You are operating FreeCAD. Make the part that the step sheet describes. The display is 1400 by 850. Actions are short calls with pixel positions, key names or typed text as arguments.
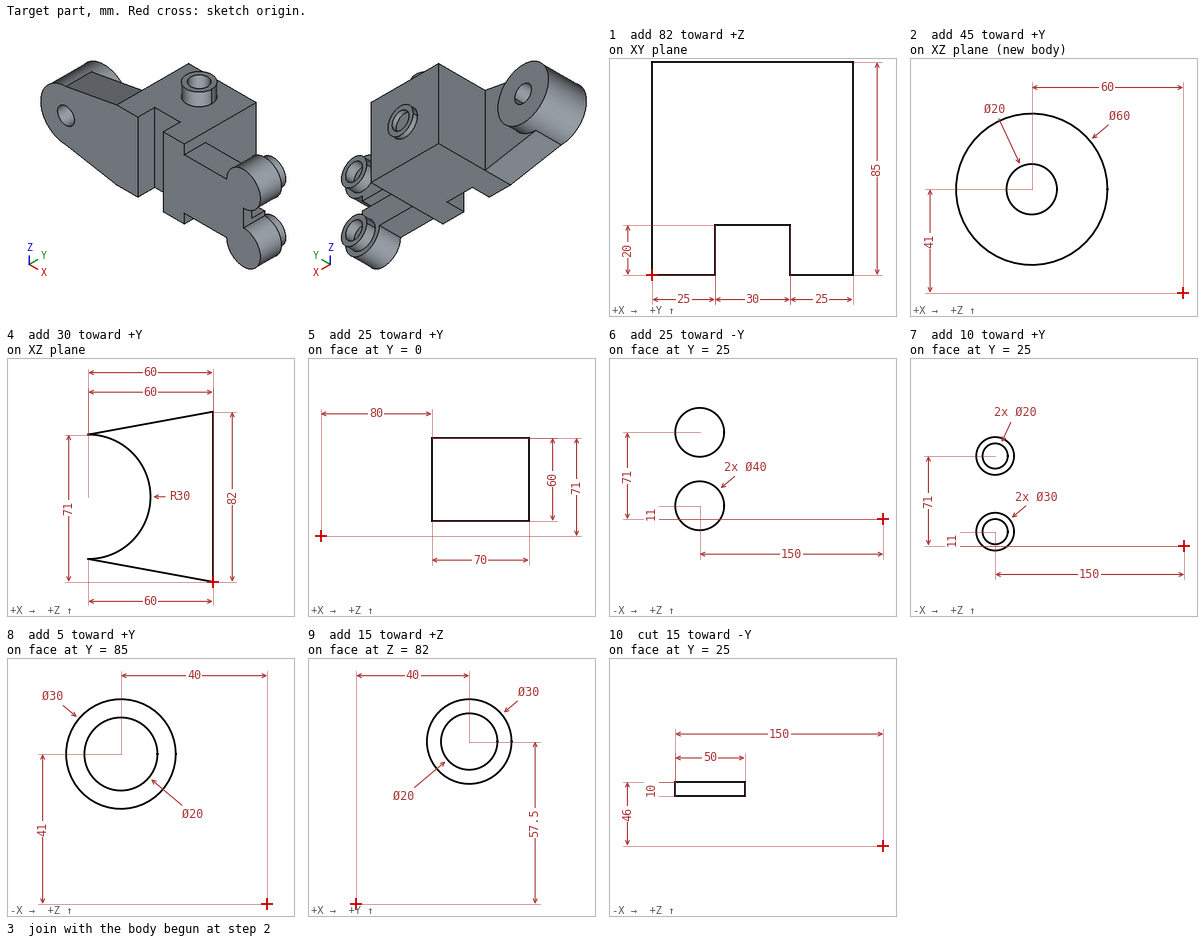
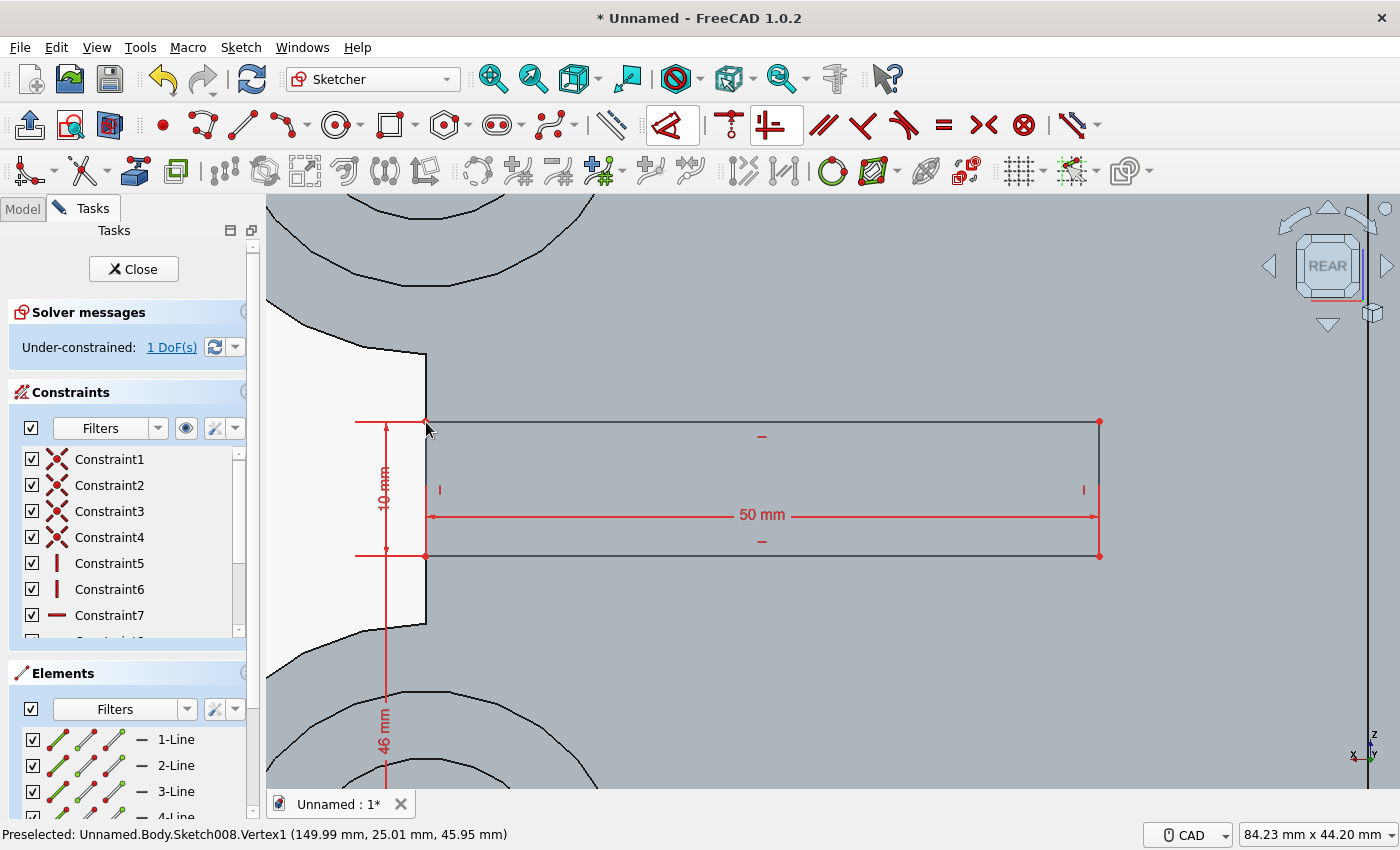
click(426, 422)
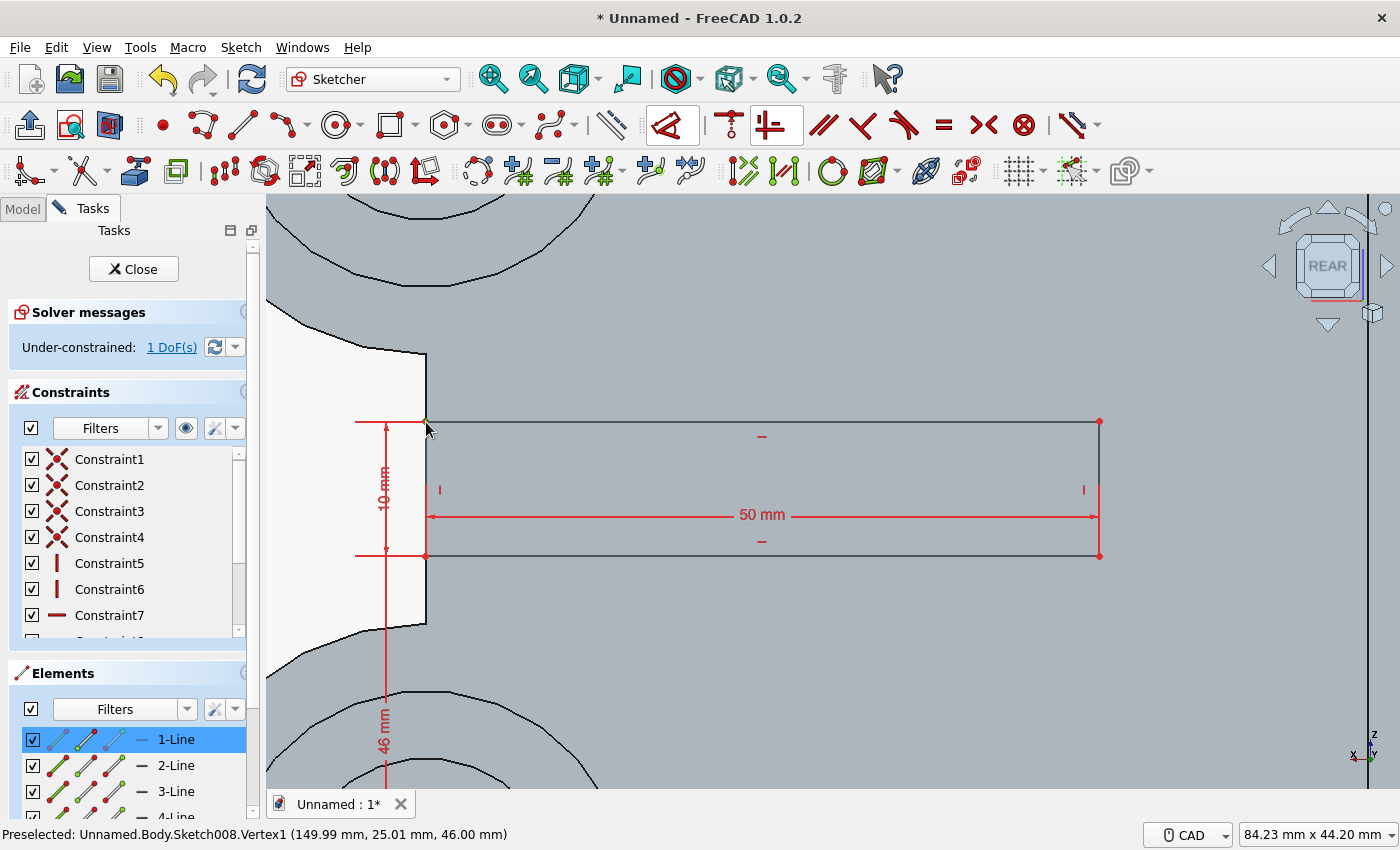
key(l)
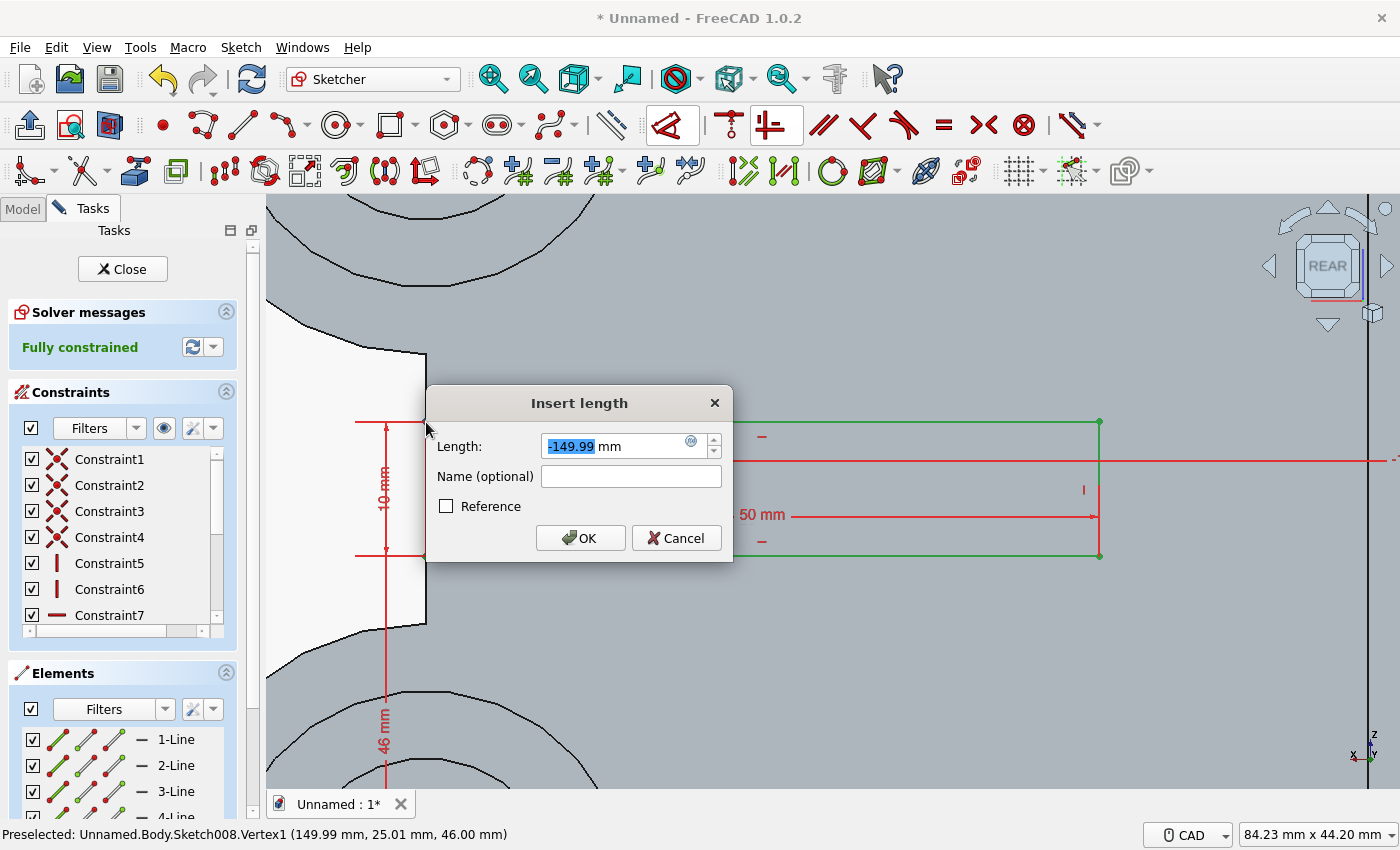
text(-150)
key(Return)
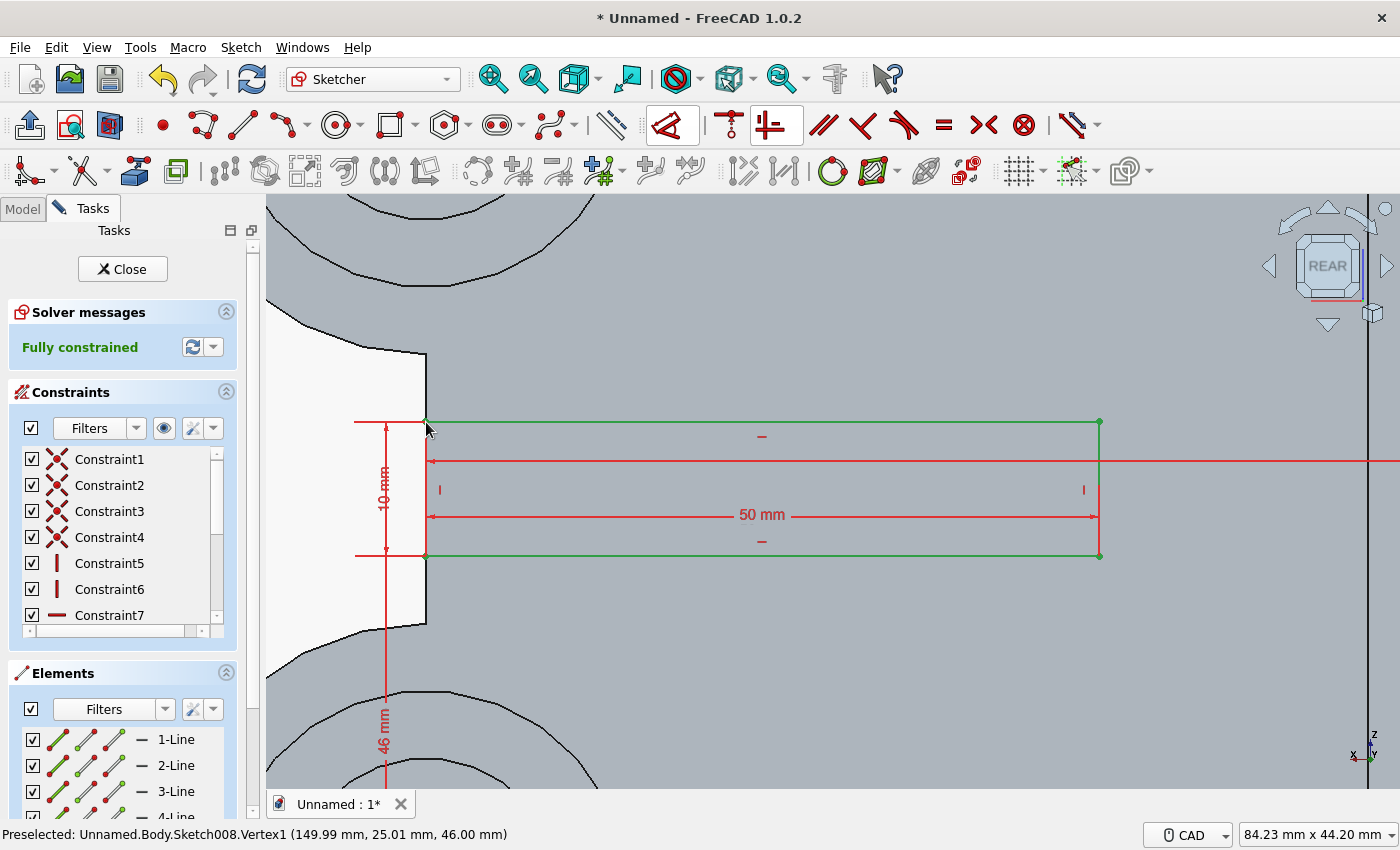
click(123, 269)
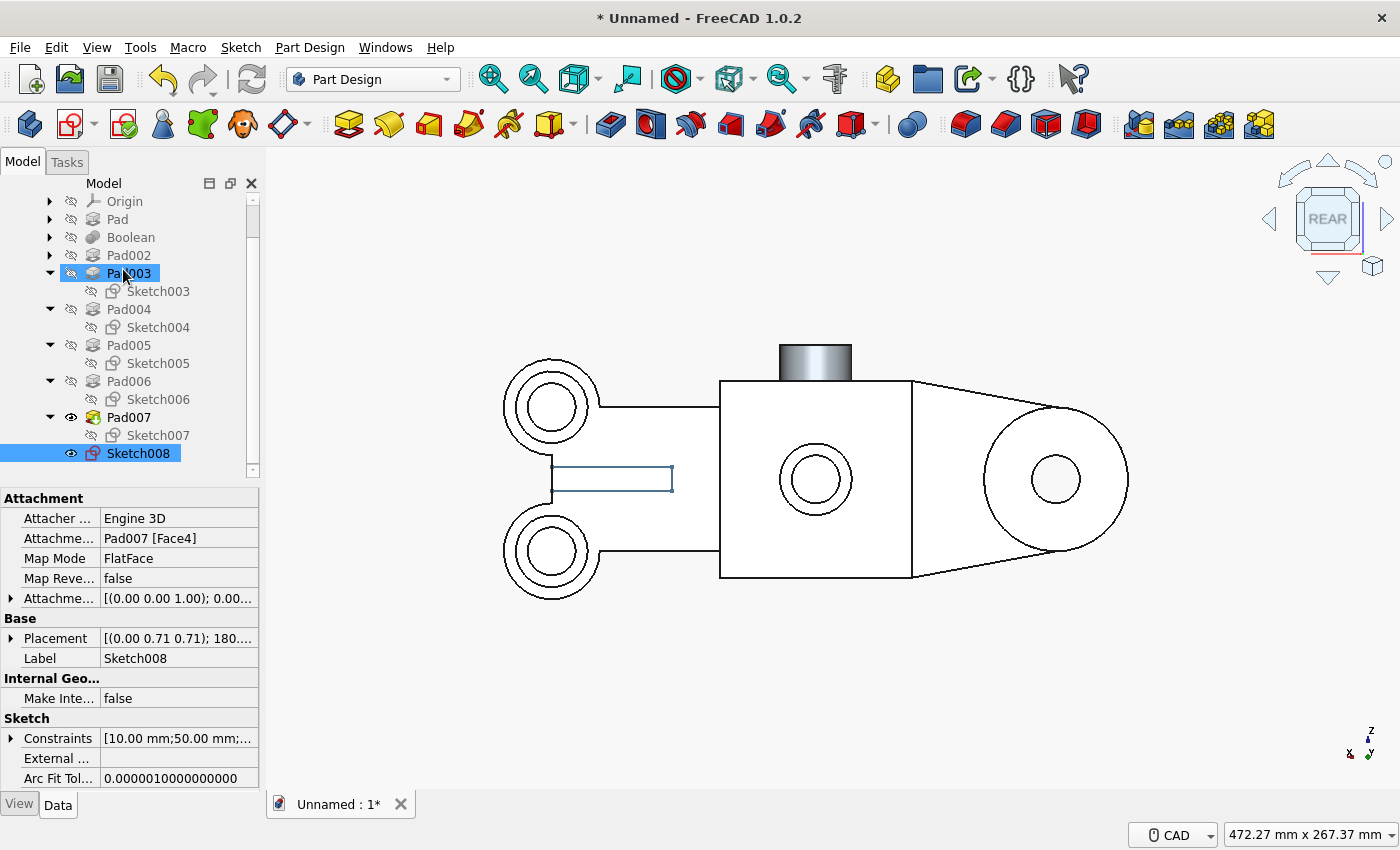
click(612, 124)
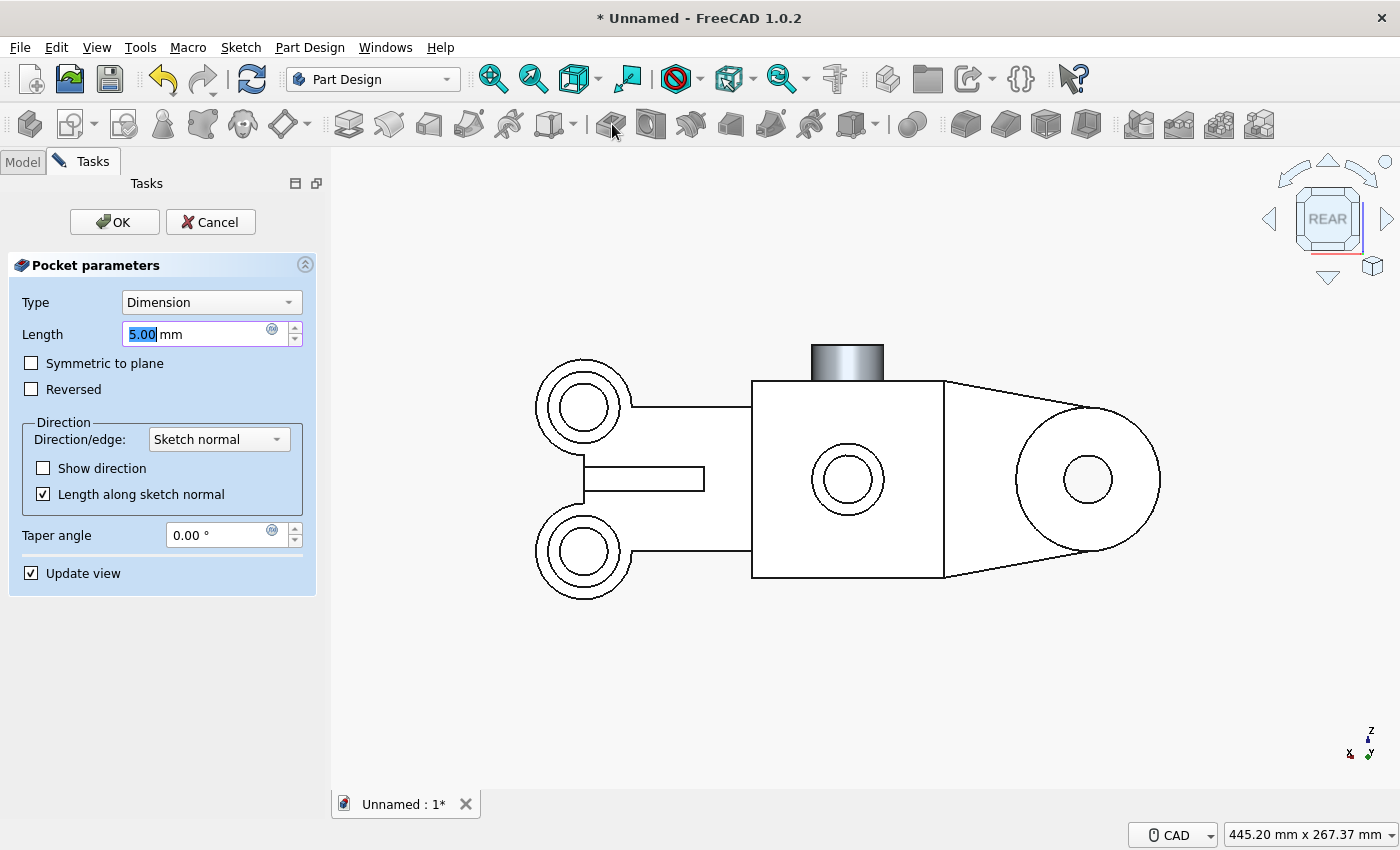
text(15)
key(Tab)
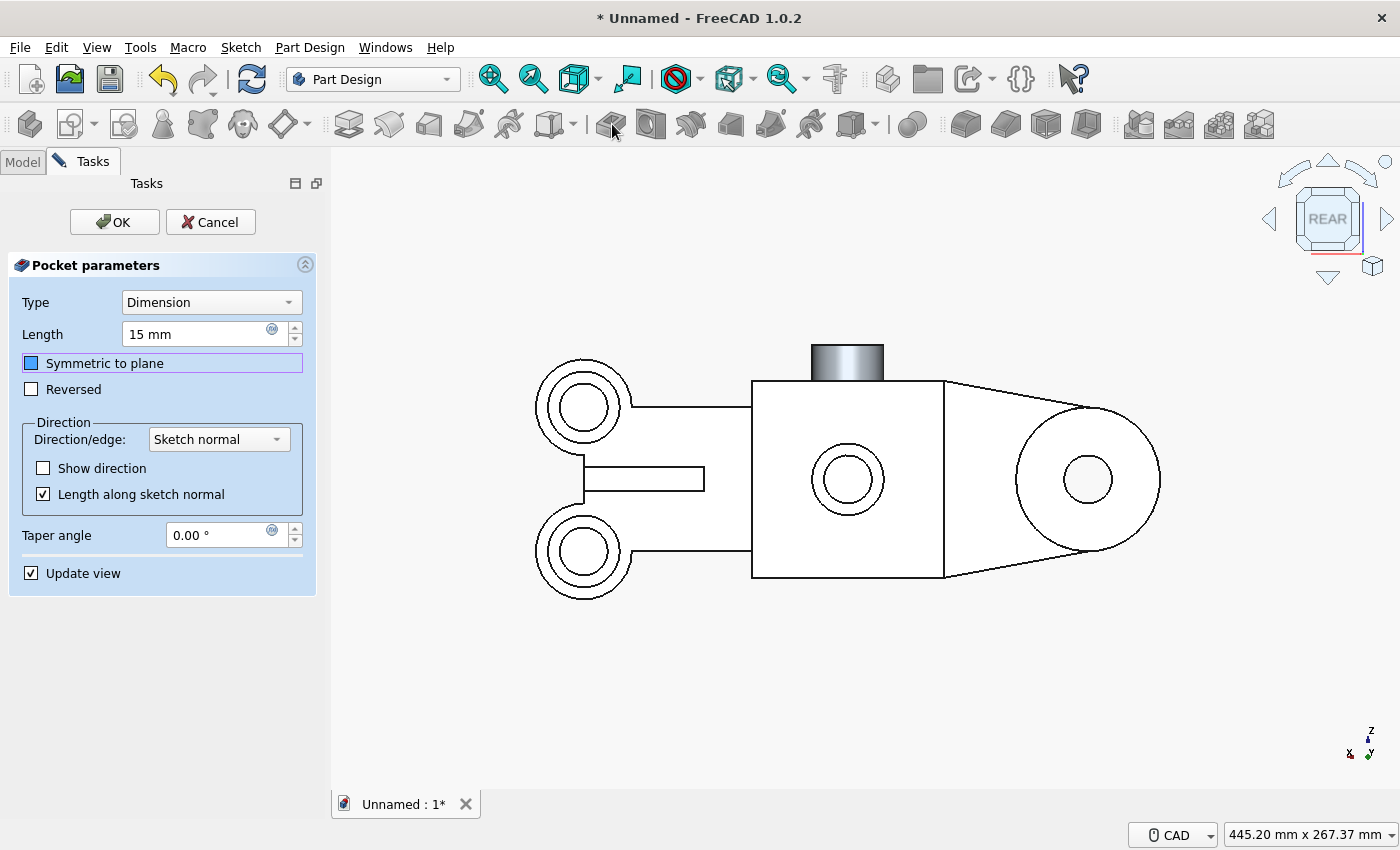
click(115, 222)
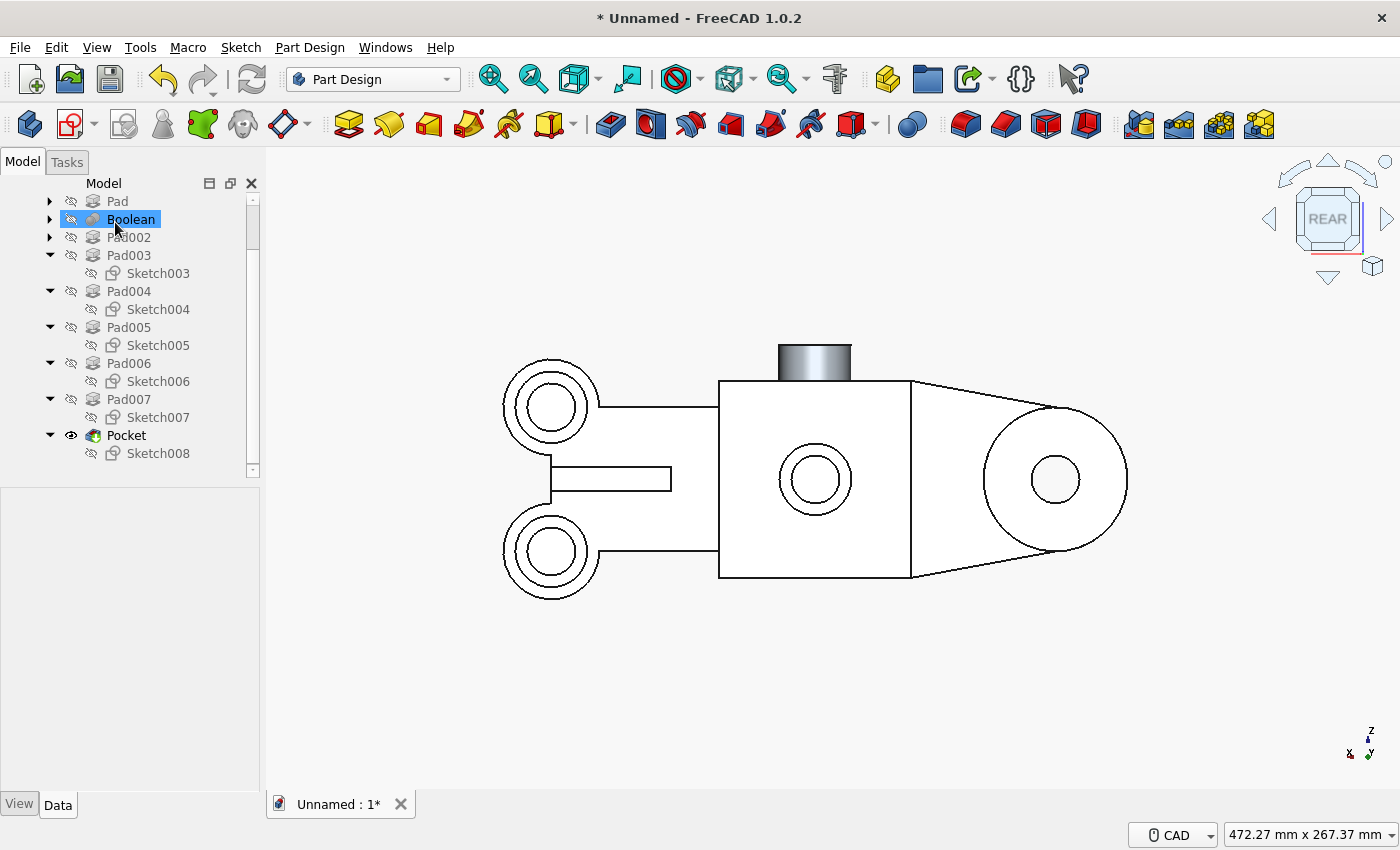
key(0)